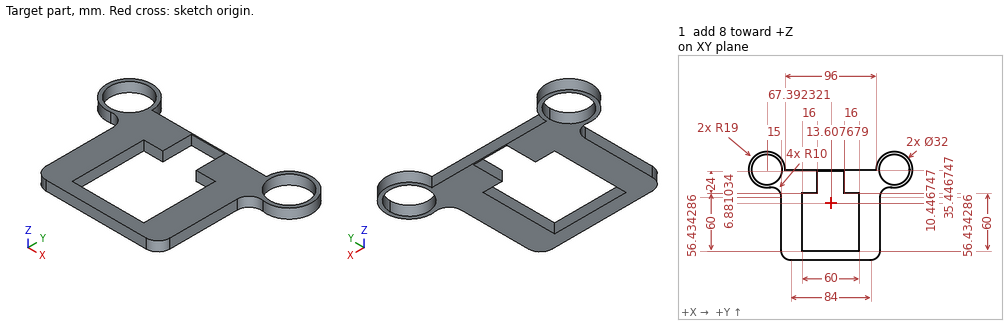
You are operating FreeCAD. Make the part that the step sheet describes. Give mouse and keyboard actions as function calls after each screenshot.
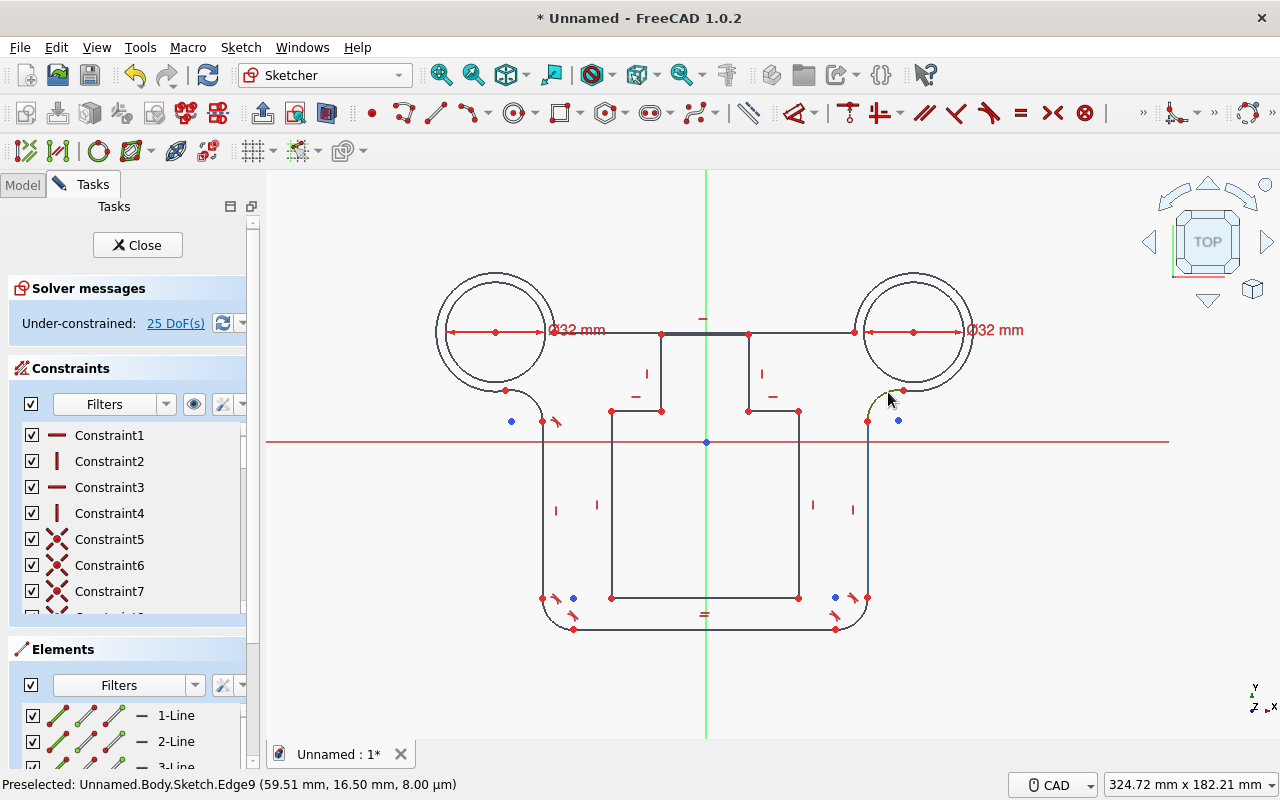
click(990, 114)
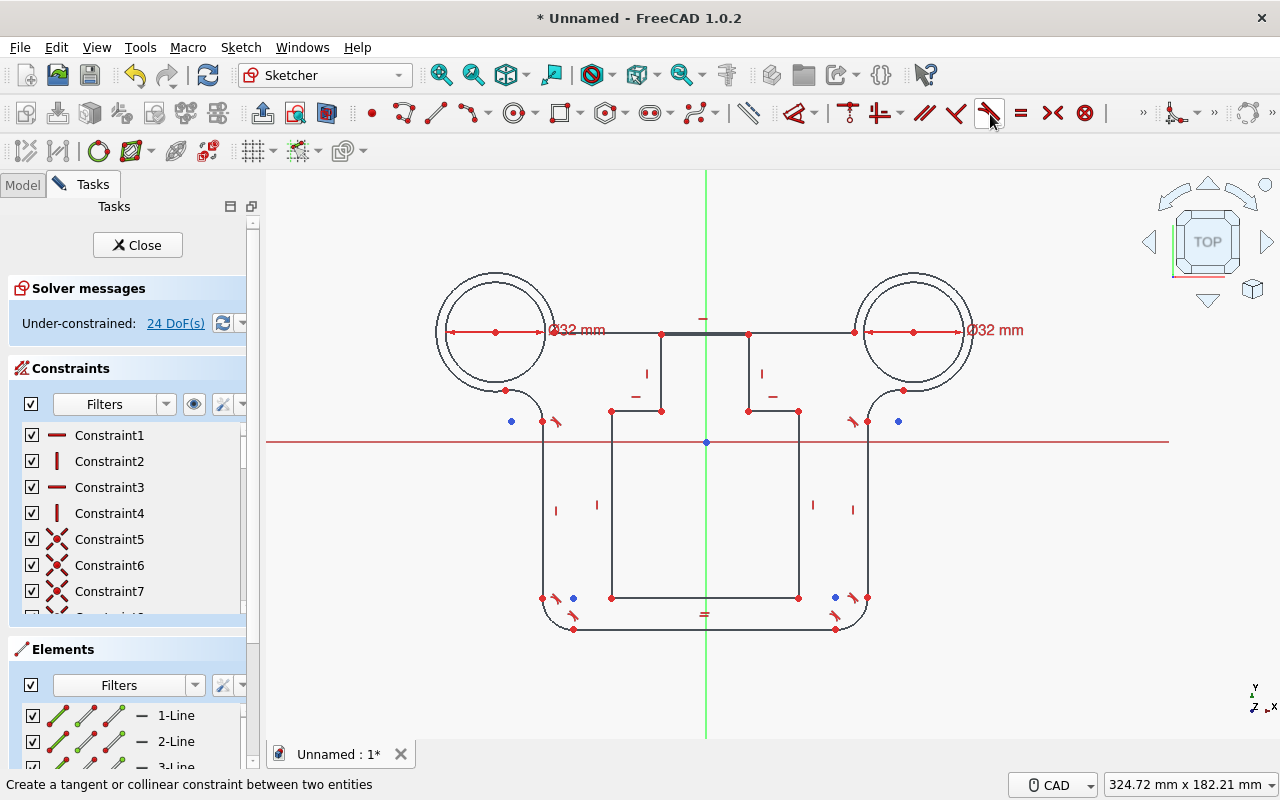
scroll(502, 273, up, 2)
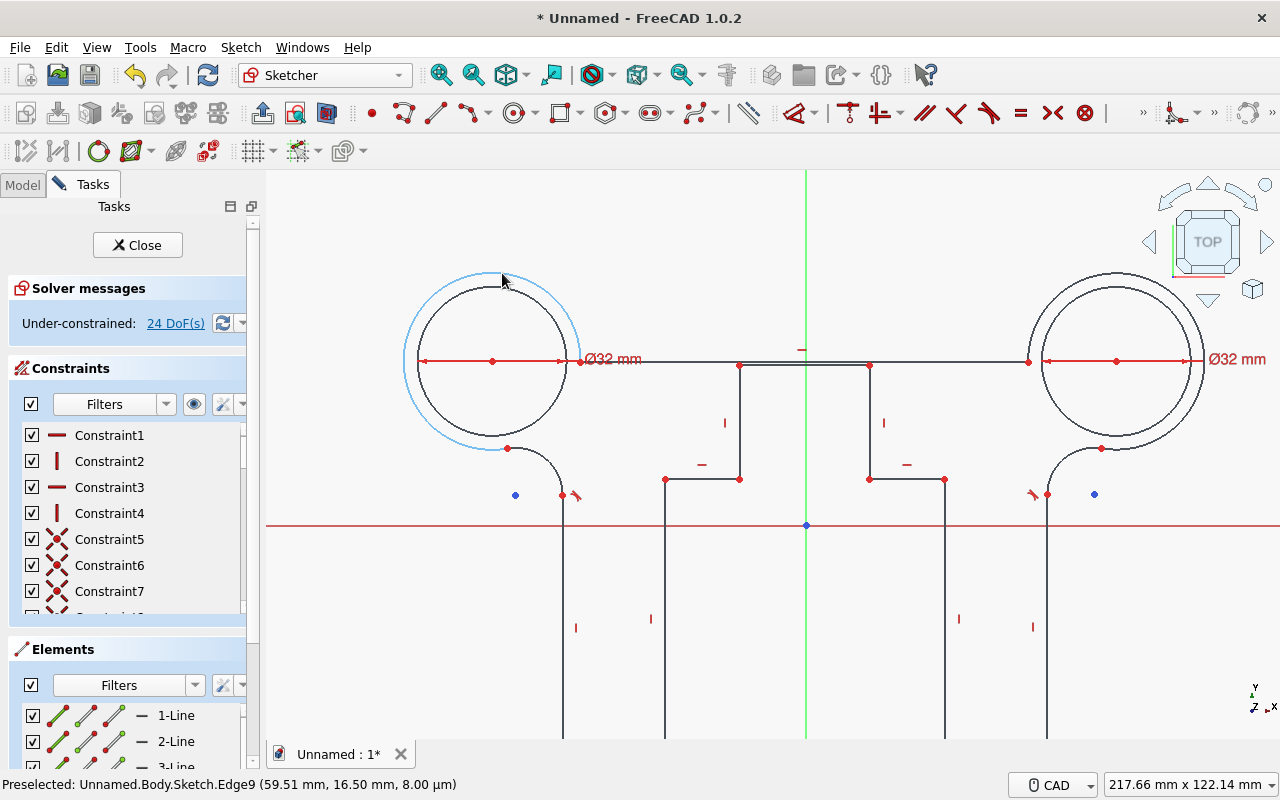
click(502, 273)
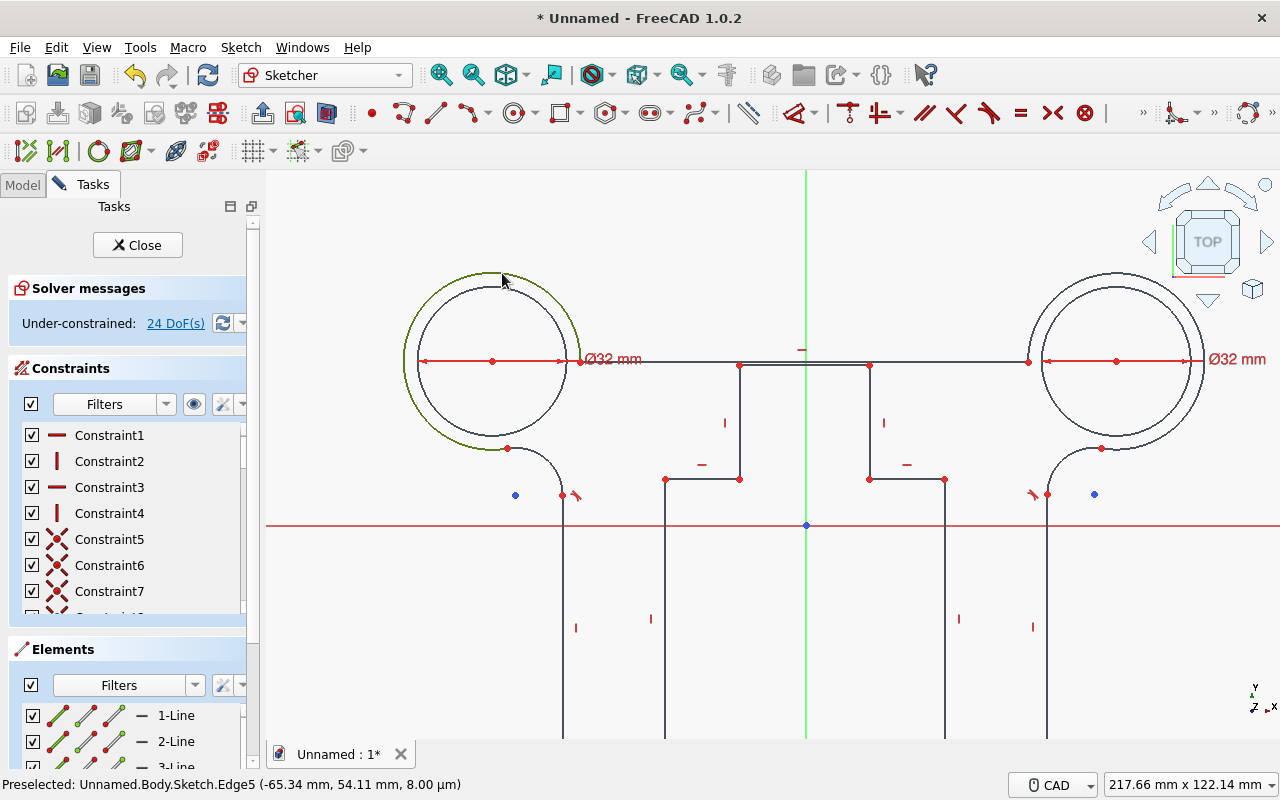
click(556, 472)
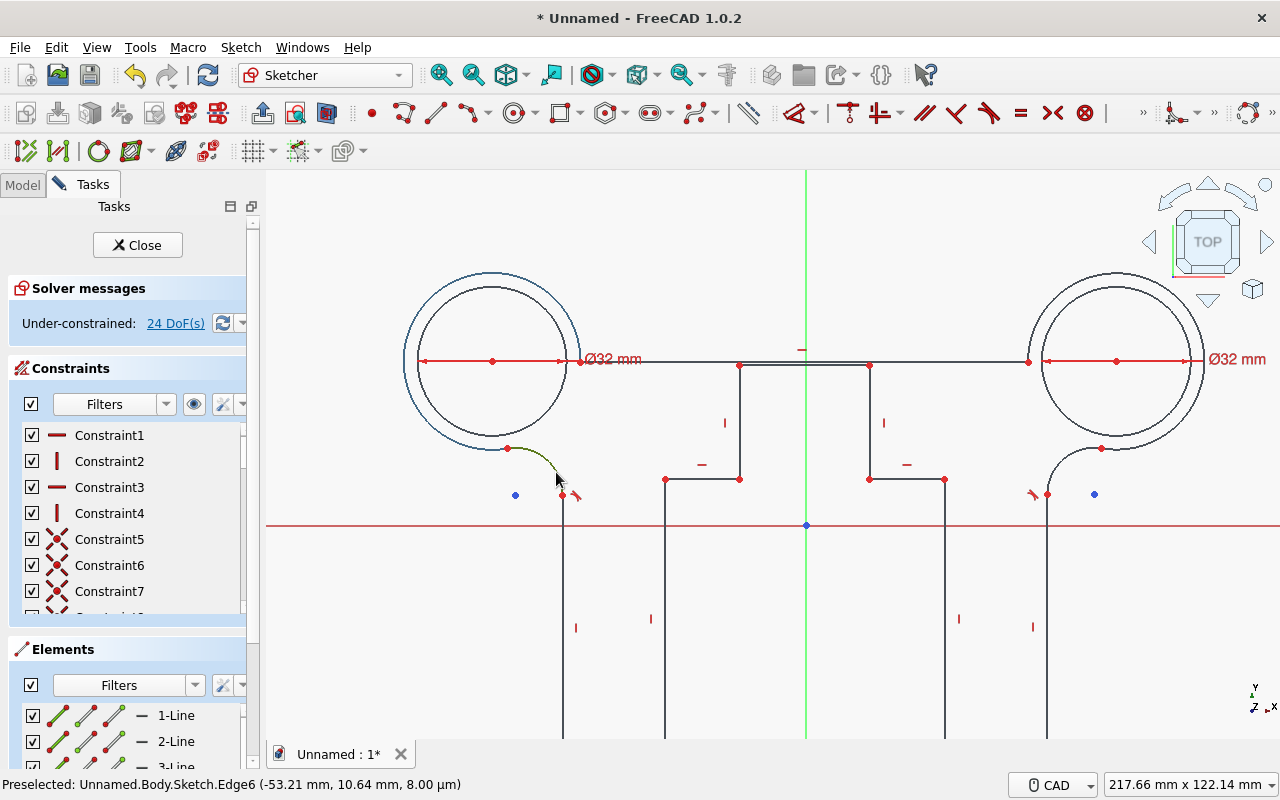
click(990, 114)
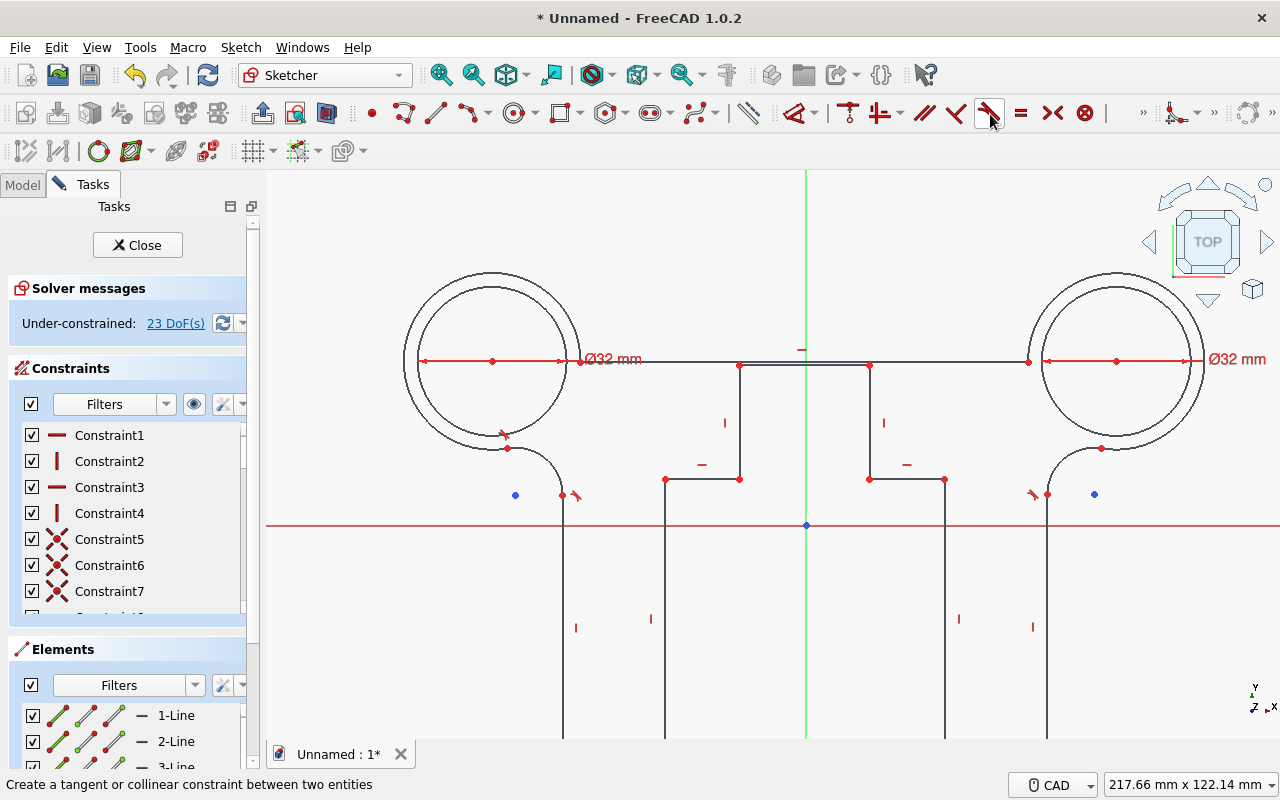
click(1078, 451)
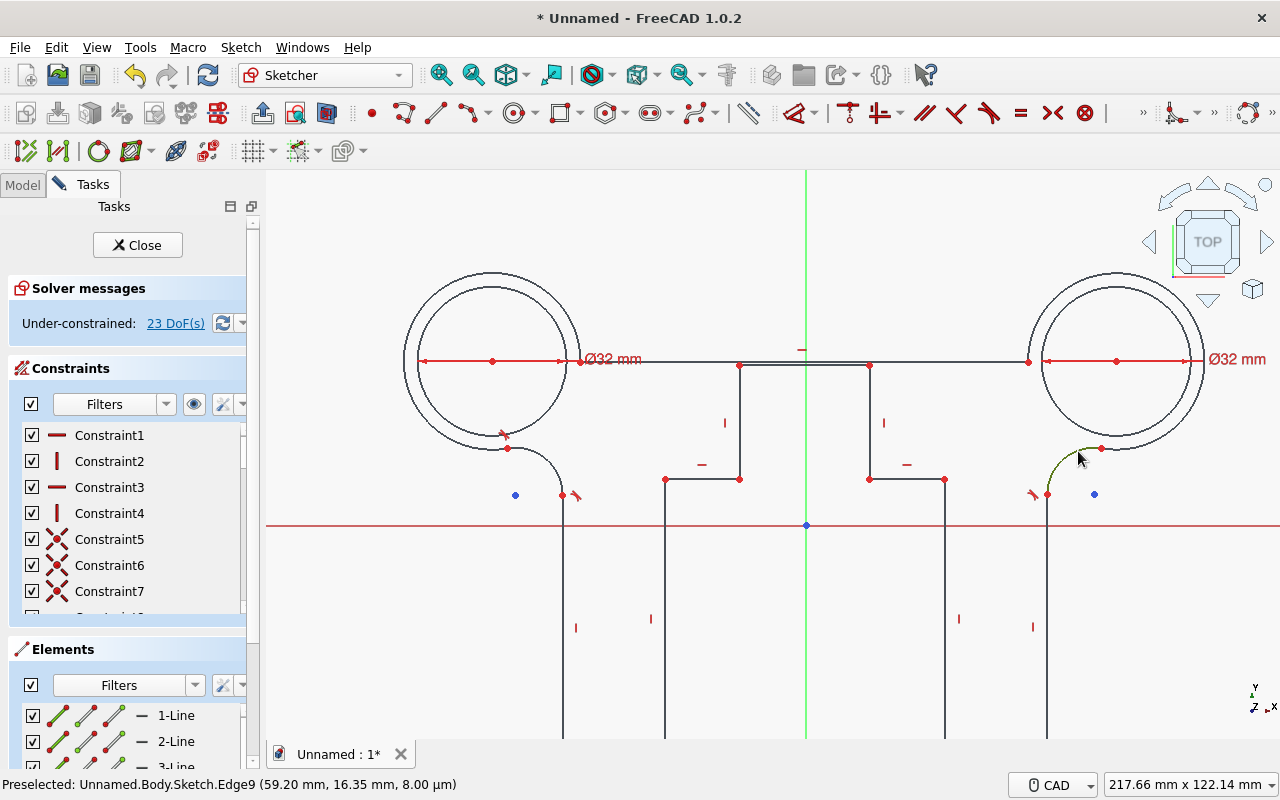
click(1106, 274)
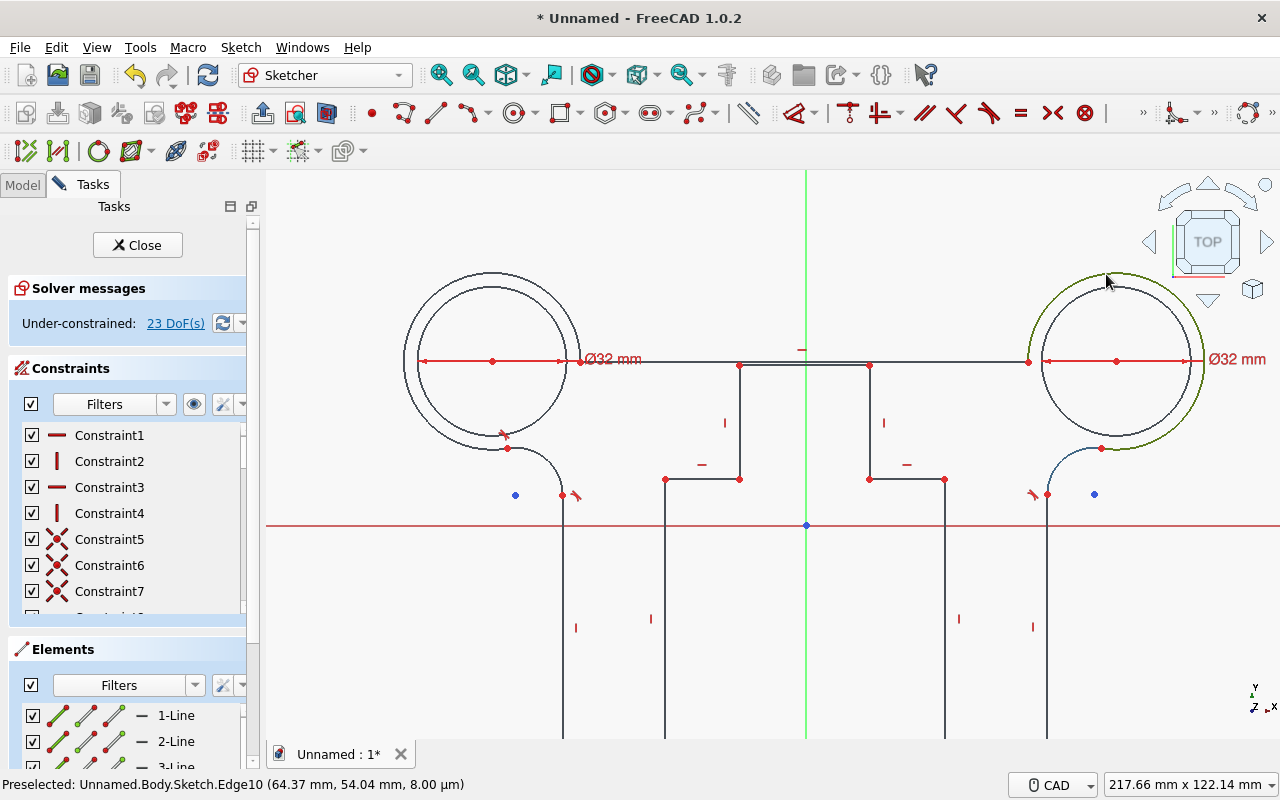
click(990, 114)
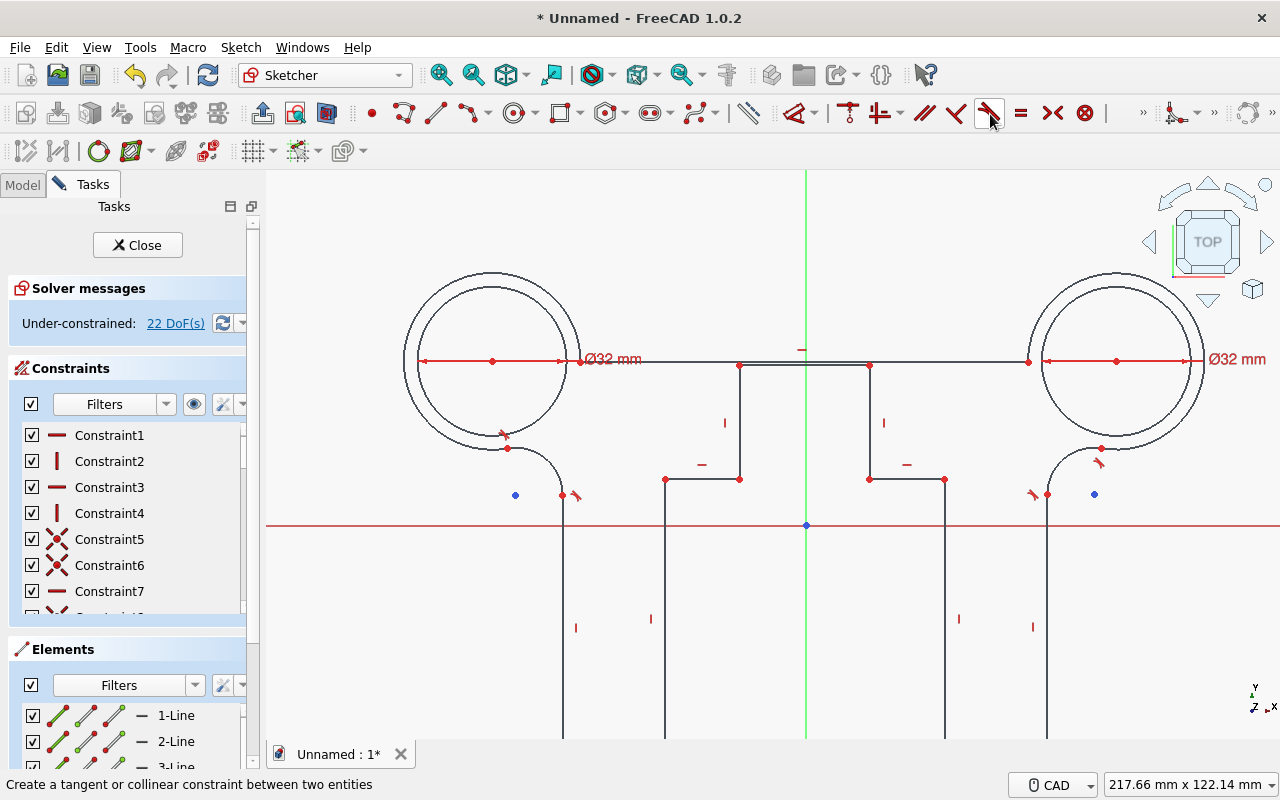
click(556, 471)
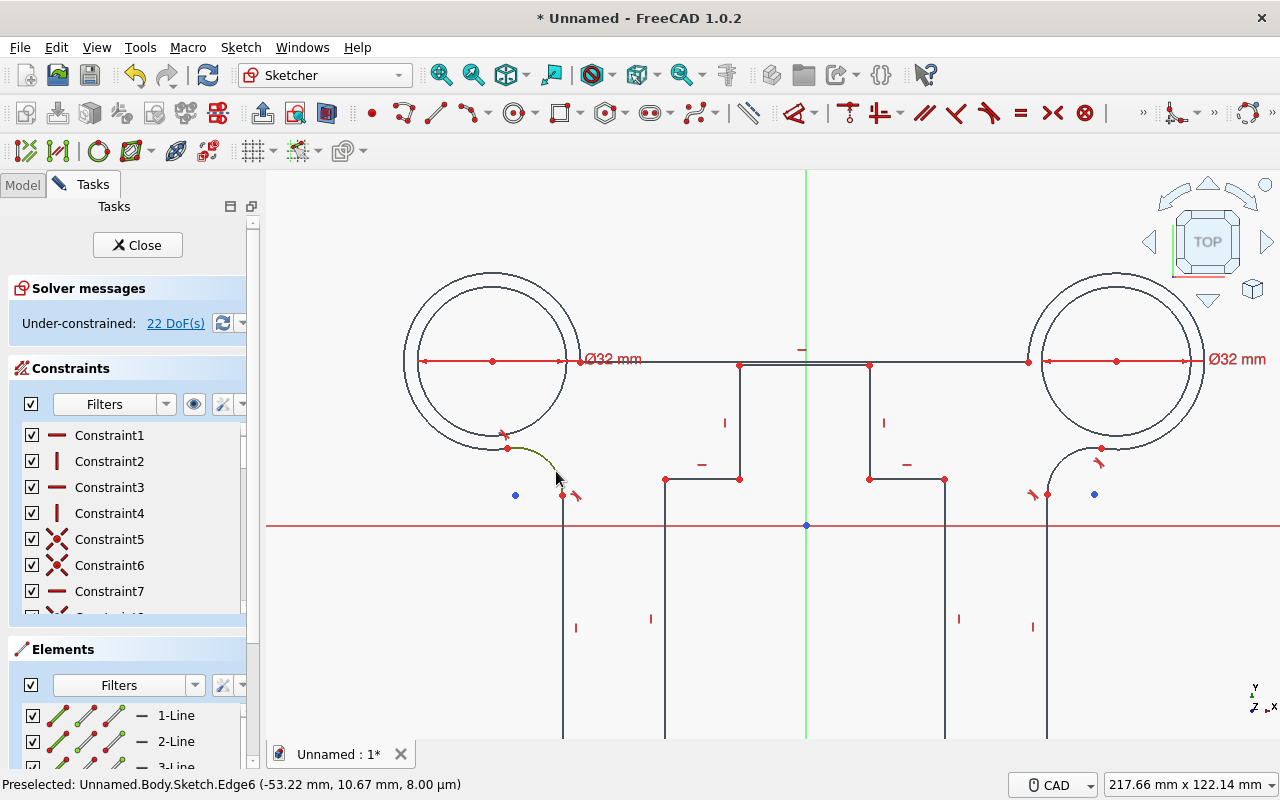
scroll(501, 272, down, 2)